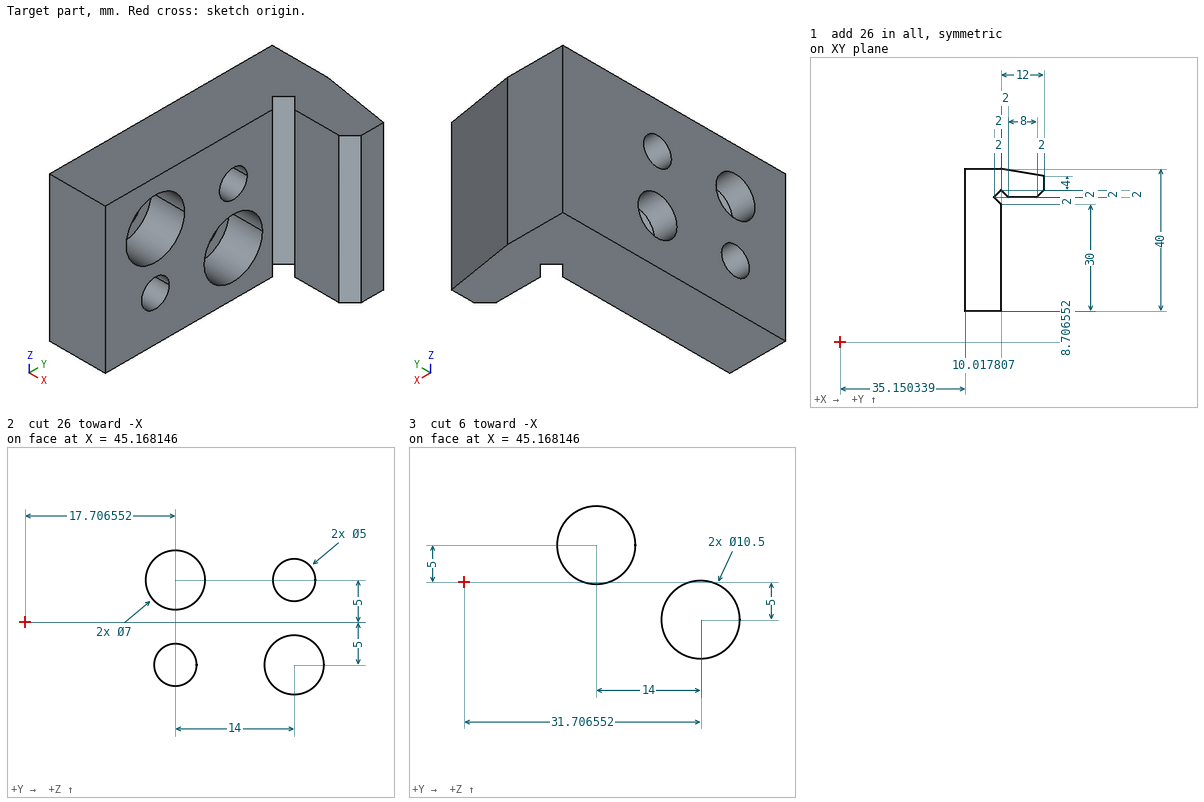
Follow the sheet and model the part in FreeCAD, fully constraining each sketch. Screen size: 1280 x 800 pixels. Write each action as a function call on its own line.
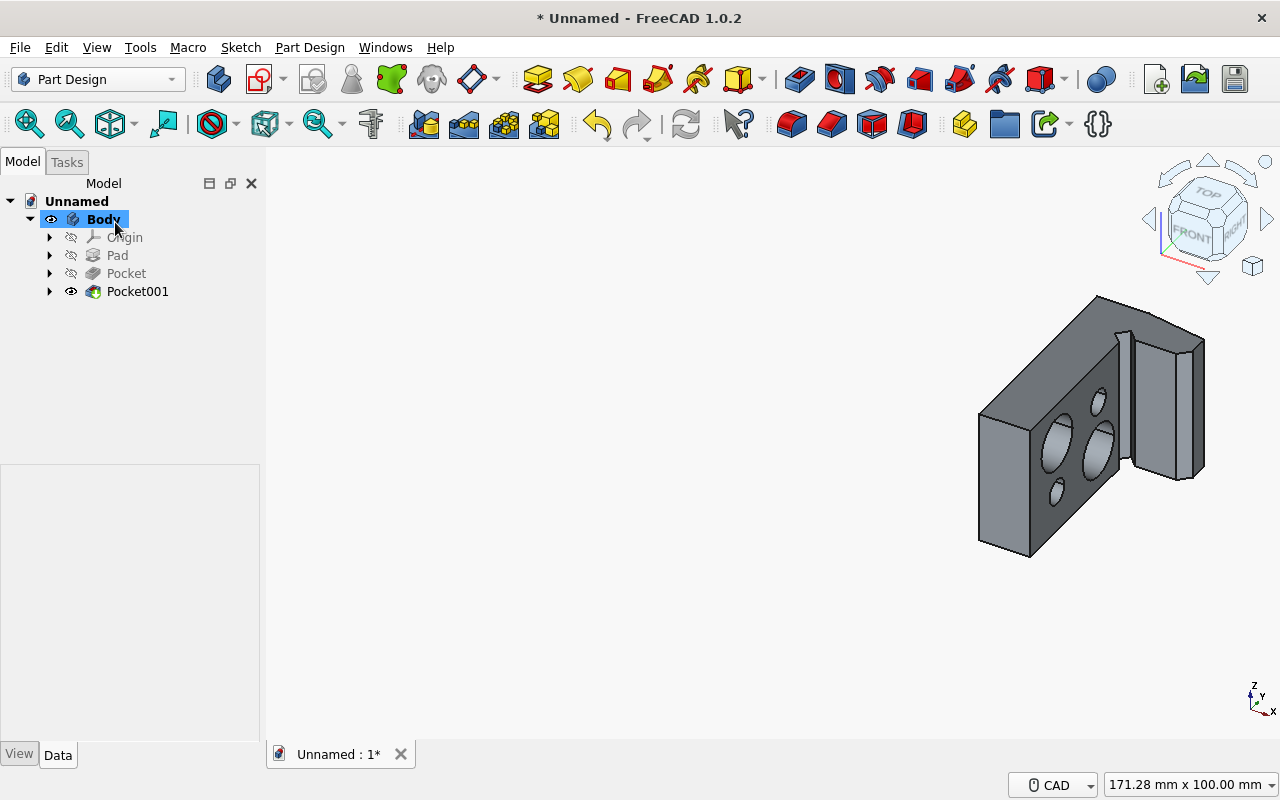
key(0)